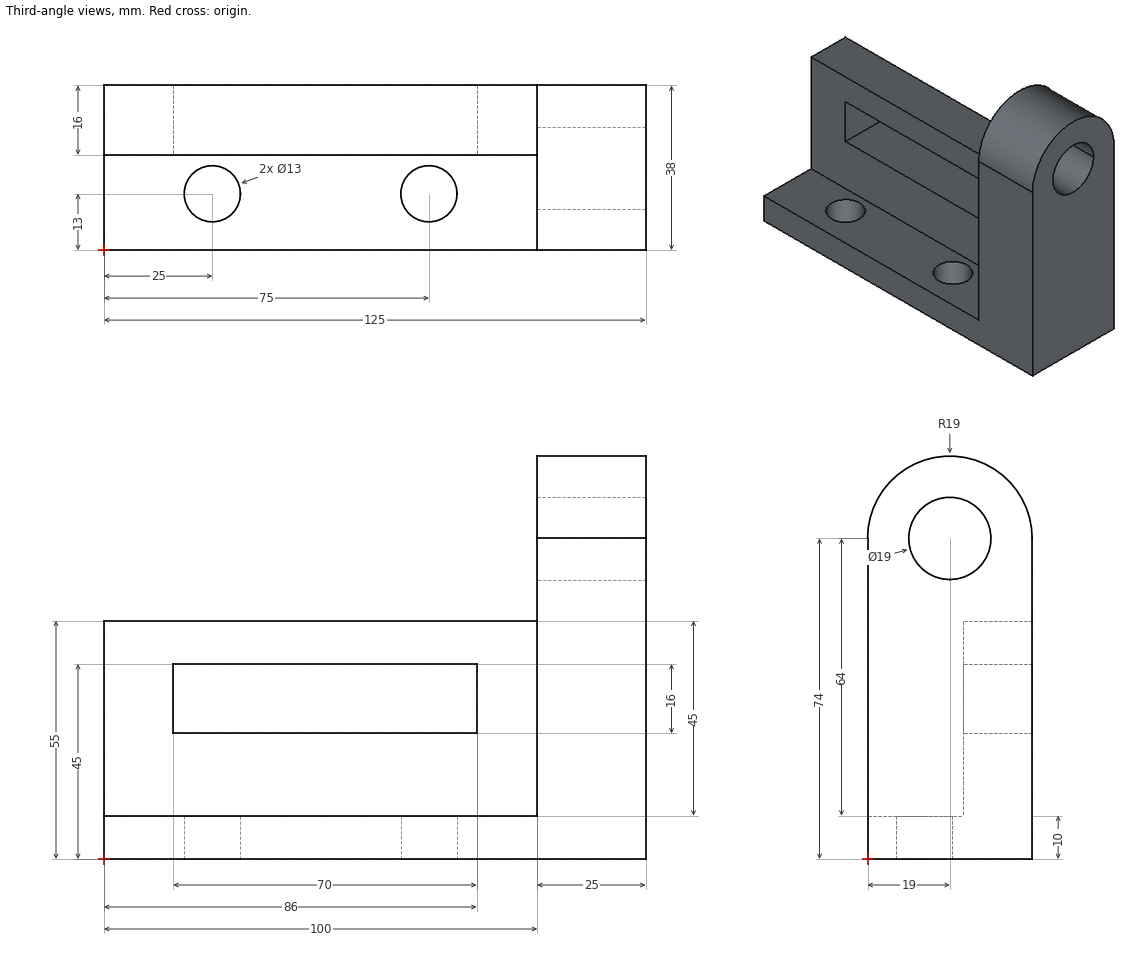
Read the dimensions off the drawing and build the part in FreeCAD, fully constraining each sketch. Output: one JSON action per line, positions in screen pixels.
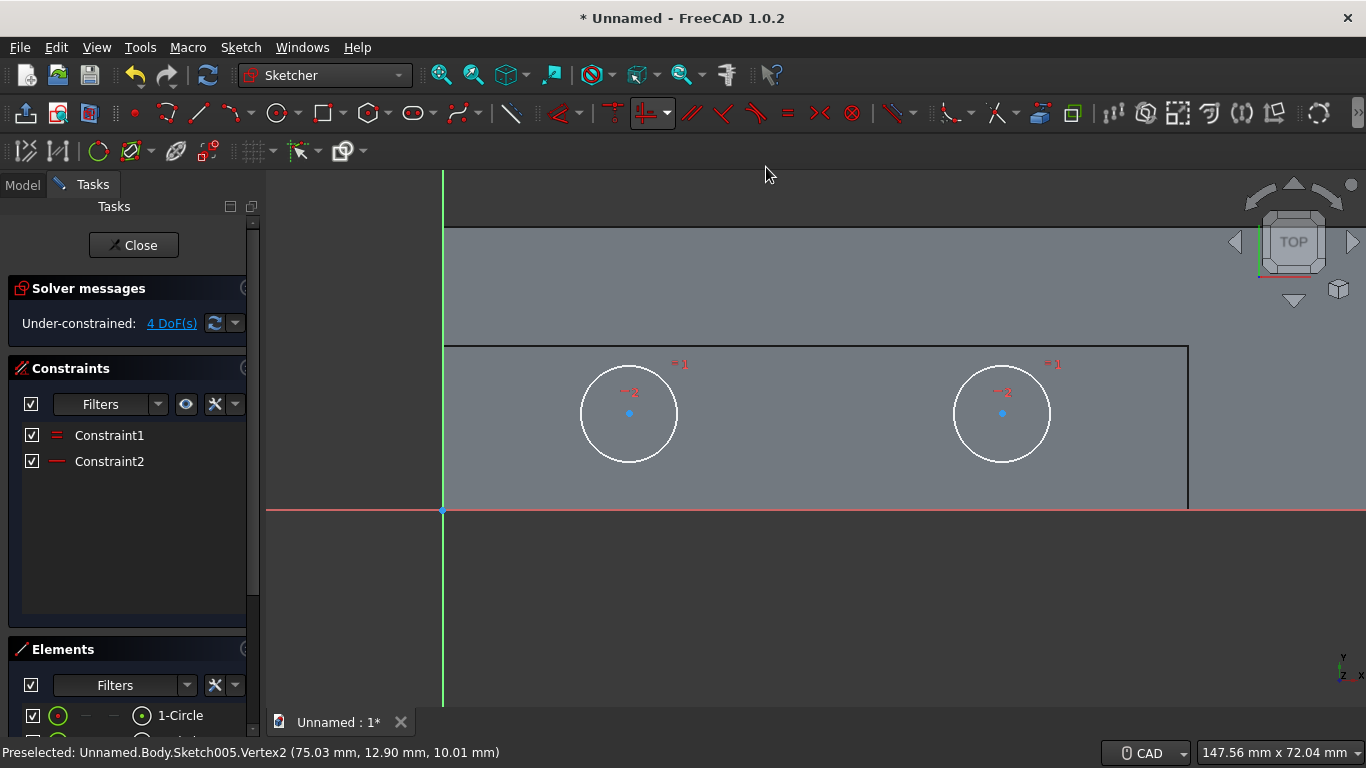
{"action": "left_click", "coordinate": [558, 114]}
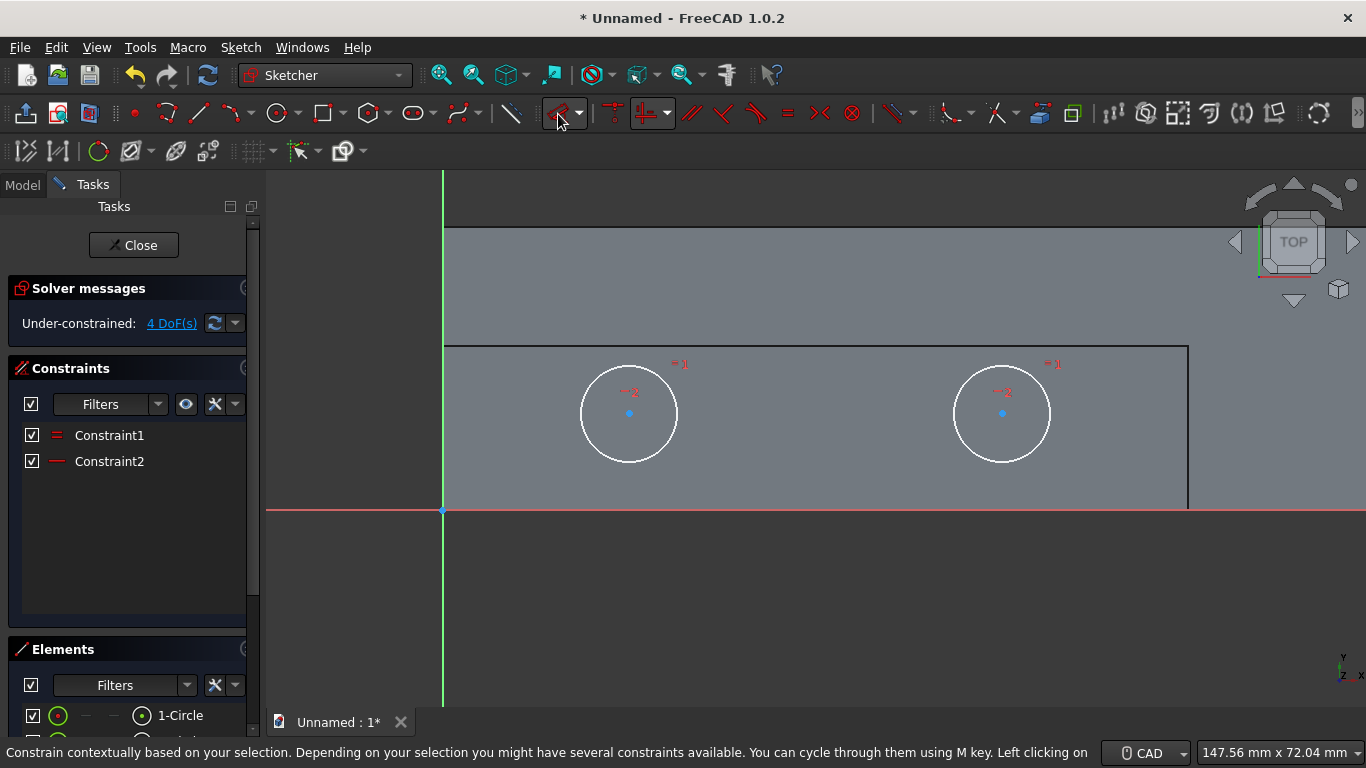
{"action": "left_click", "coordinate": [663, 380]}
{"action": "left_click", "coordinate": [686, 357]}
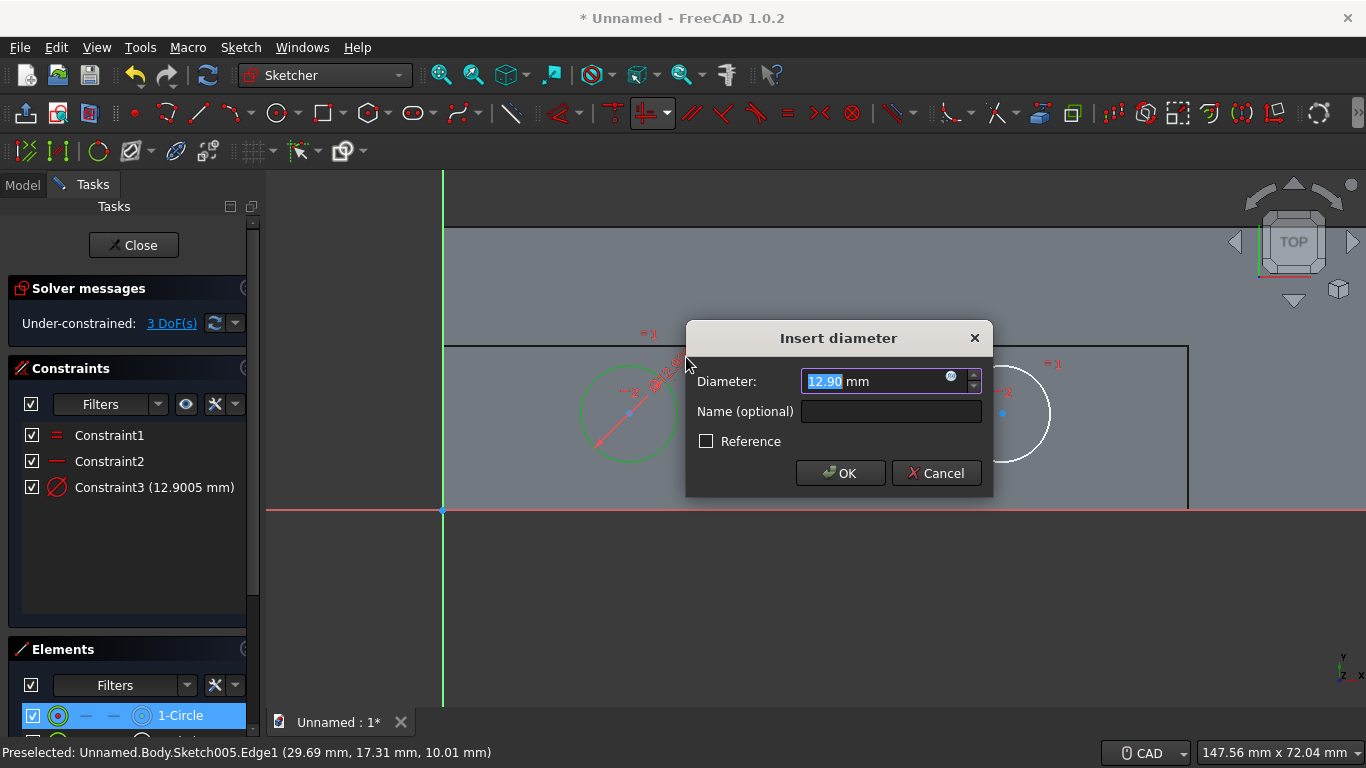
{"action": "type", "text": "13"}
{"action": "key", "text": "Return"}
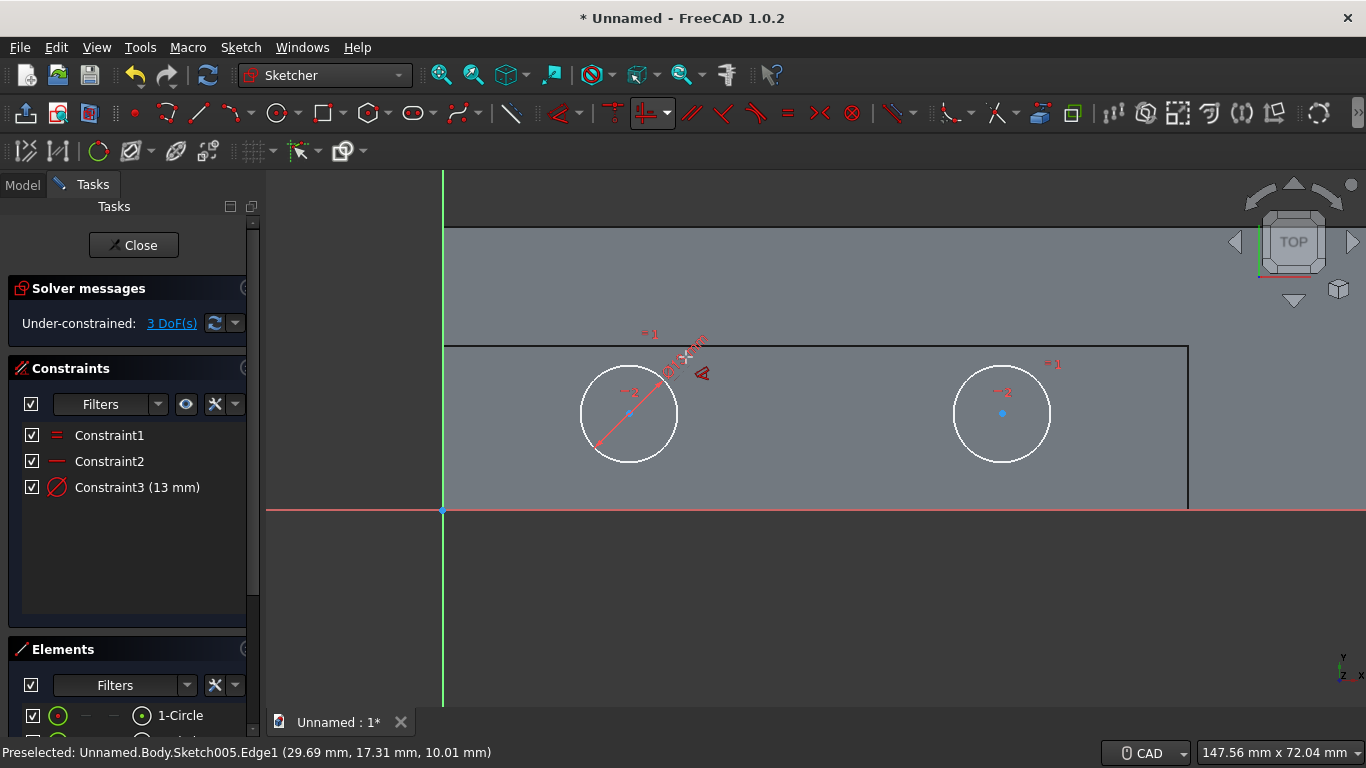
{"action": "left_click", "coordinate": [629, 414]}
{"action": "left_click", "coordinate": [536, 544]}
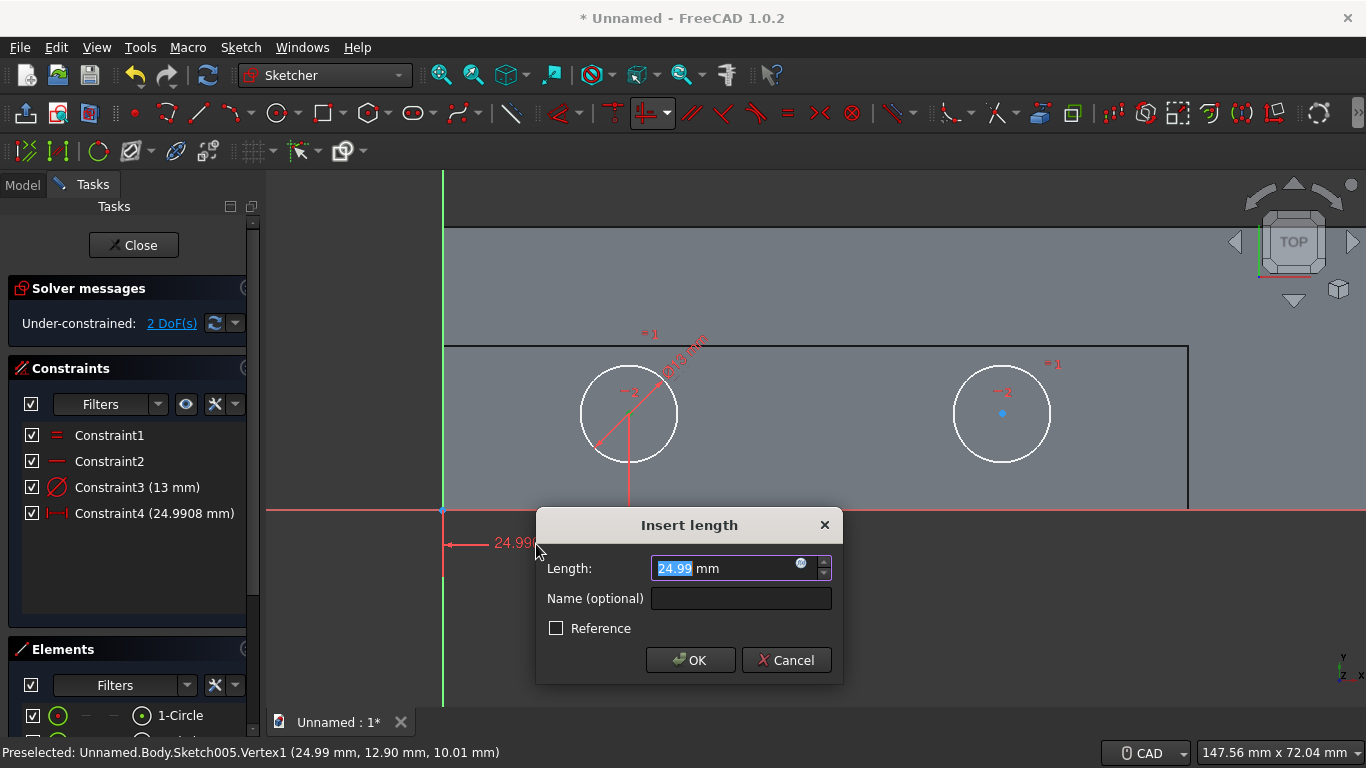
{"action": "type", "text": "25"}
{"action": "key", "text": "Return"}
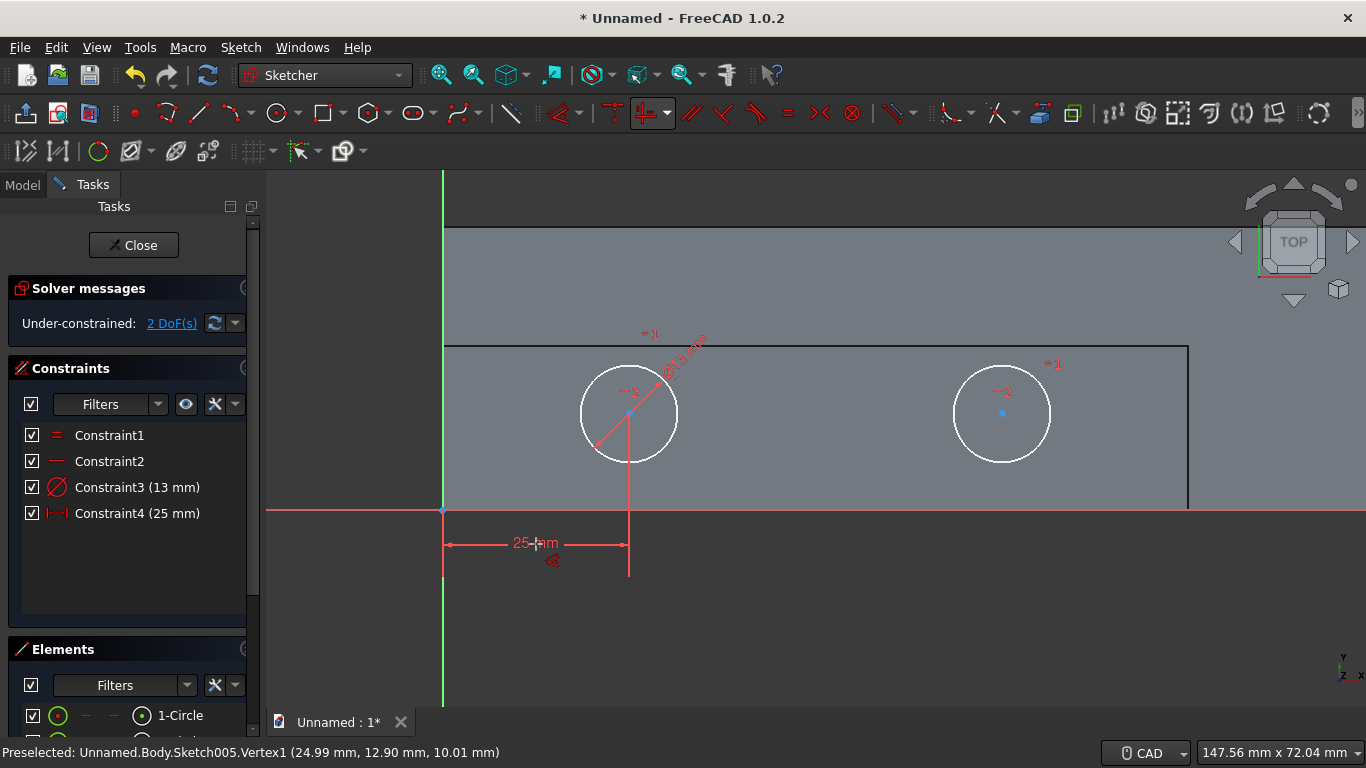
{"action": "left_click", "coordinate": [629, 414]}
{"action": "left_click", "coordinate": [409, 462]}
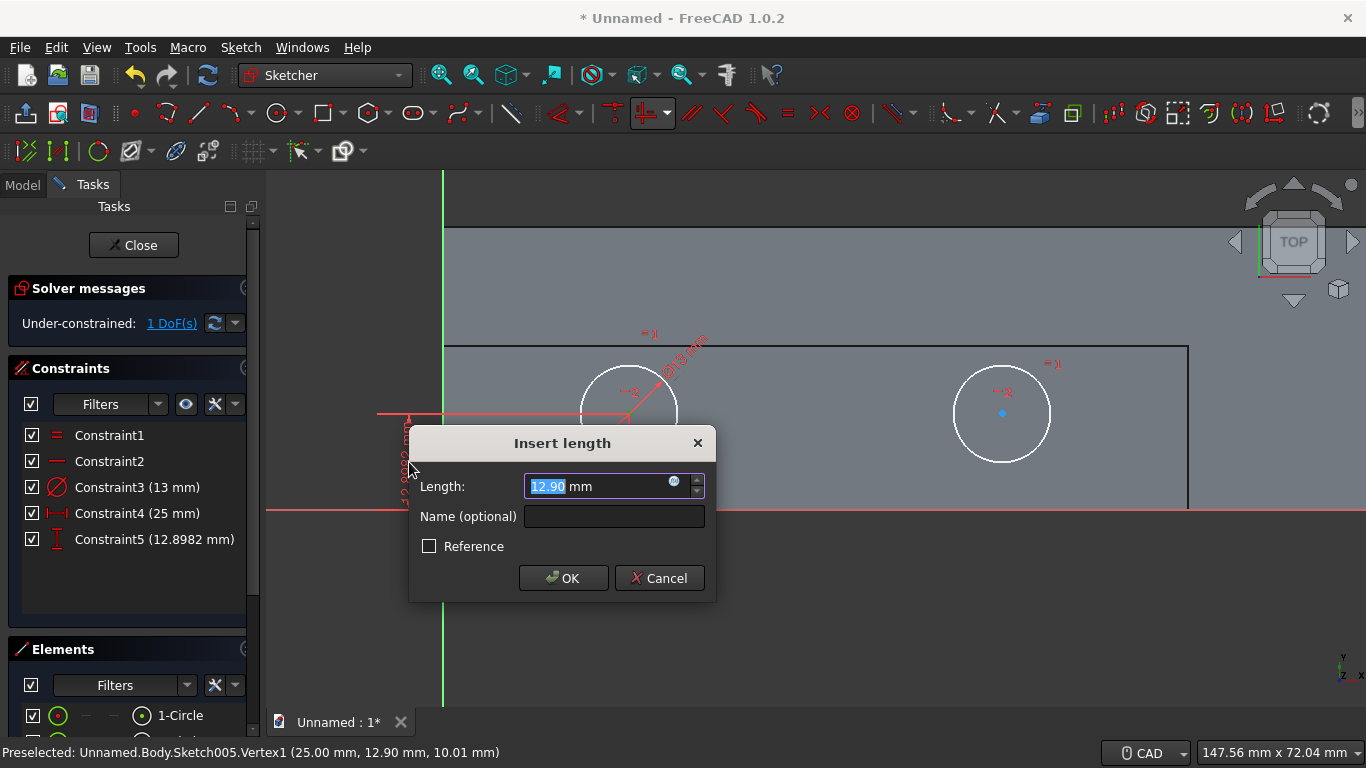
{"action": "type", "text": "13"}
{"action": "key", "text": "Return"}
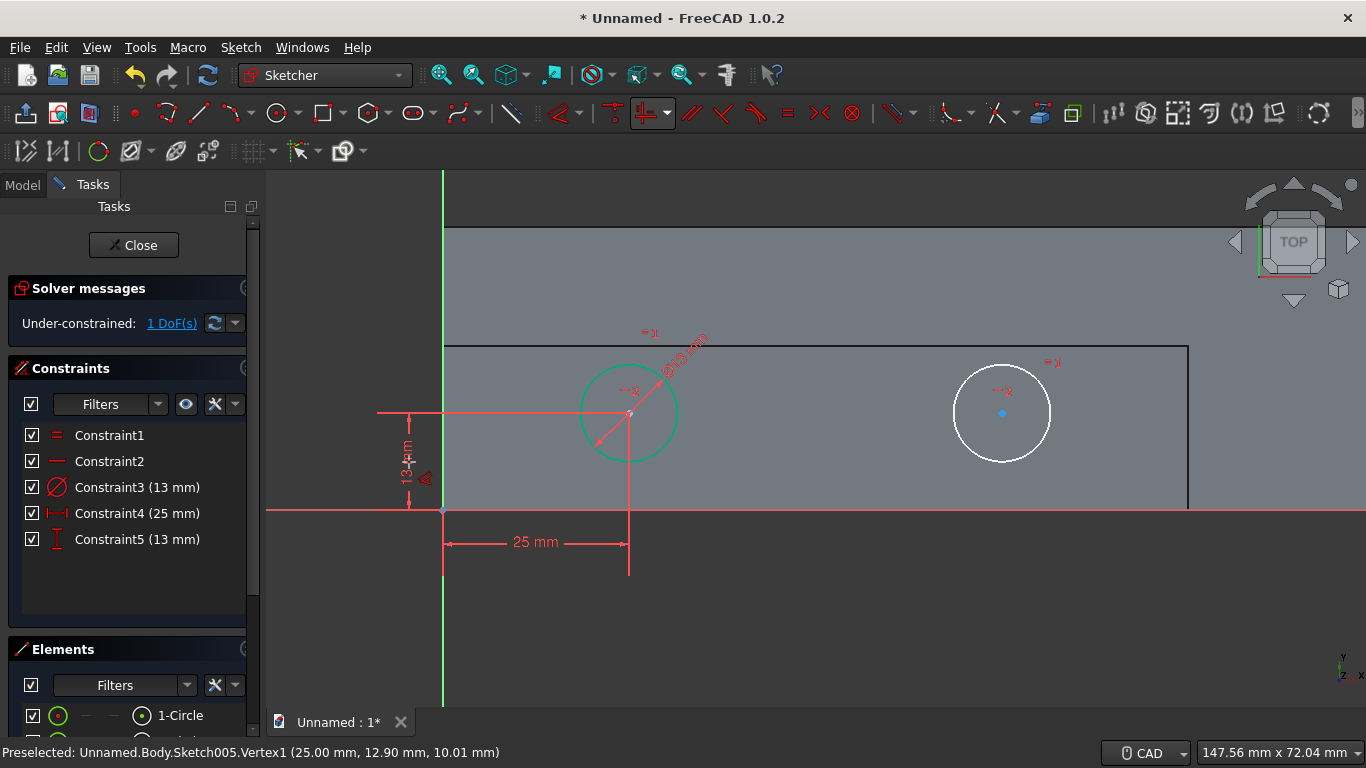
{"action": "left_click", "coordinate": [1002, 413]}
{"action": "left_click", "coordinate": [722, 544]}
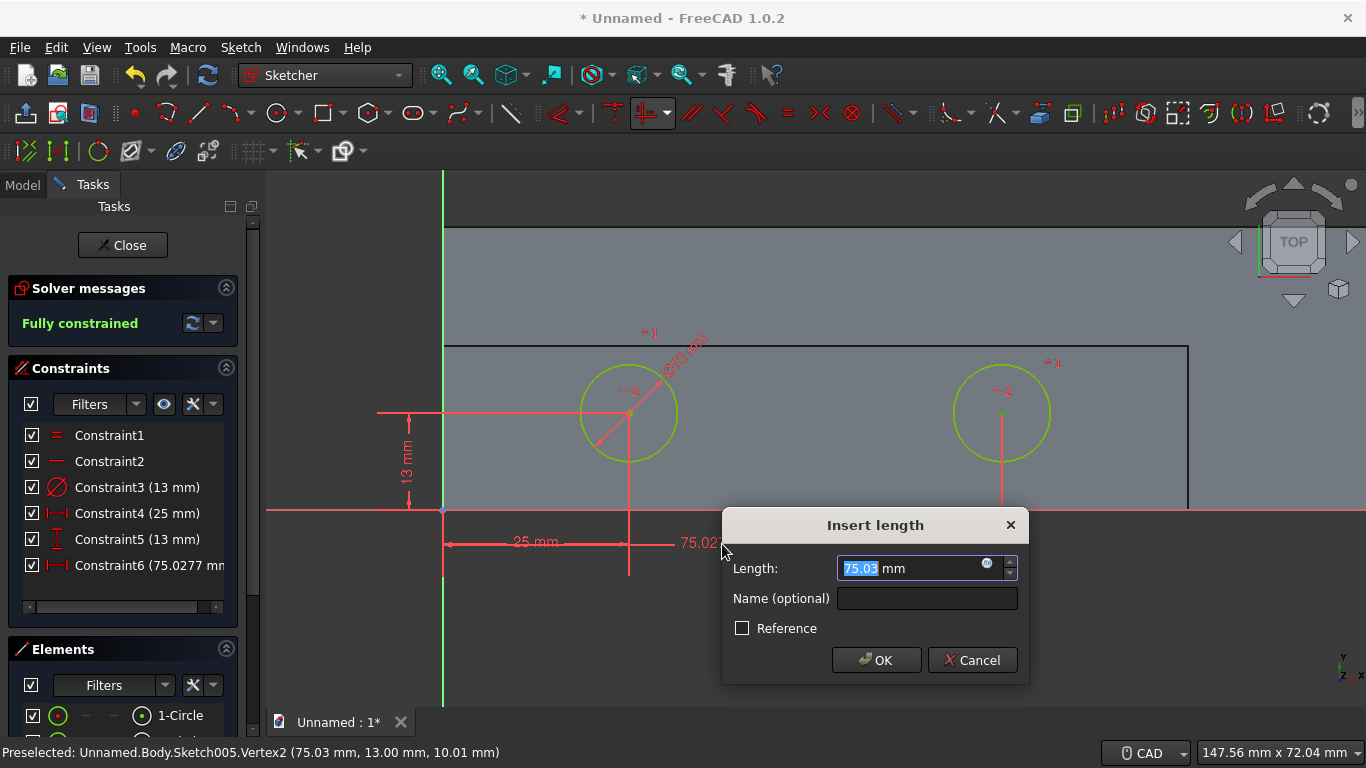
{"action": "type", "text": "75"}
{"action": "key", "text": "Return"}
{"action": "key", "text": "Escape"}